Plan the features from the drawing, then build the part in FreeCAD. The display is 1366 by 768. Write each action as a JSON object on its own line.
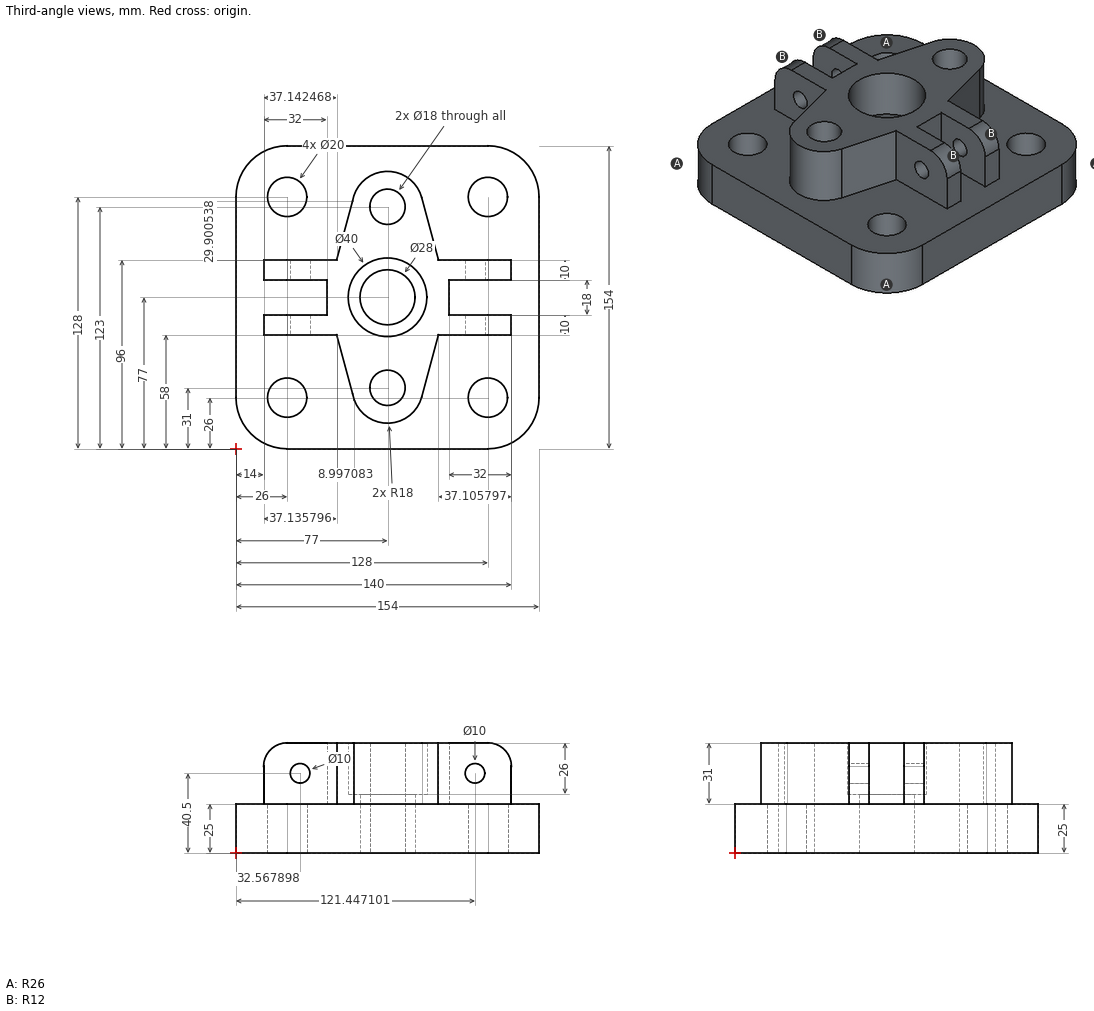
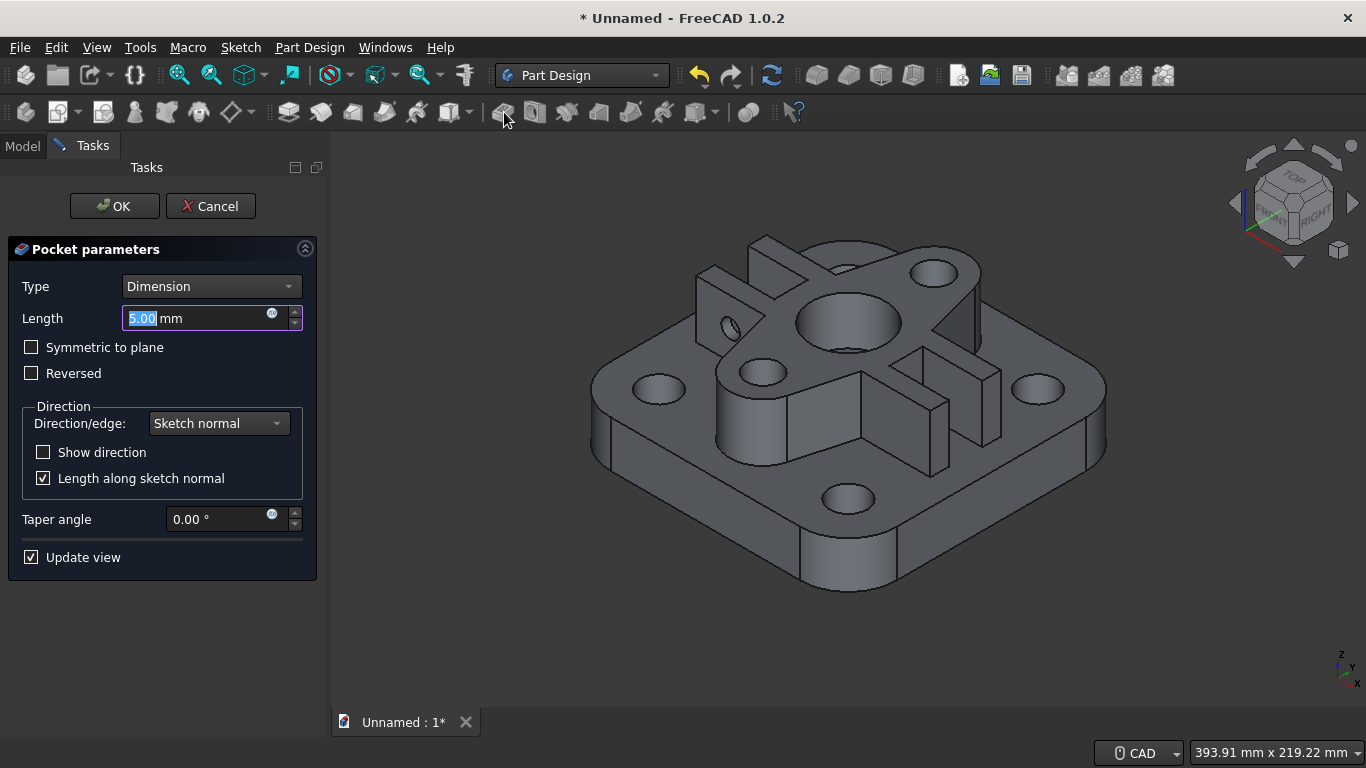
{"action": "left_click", "coordinate": [212, 286]}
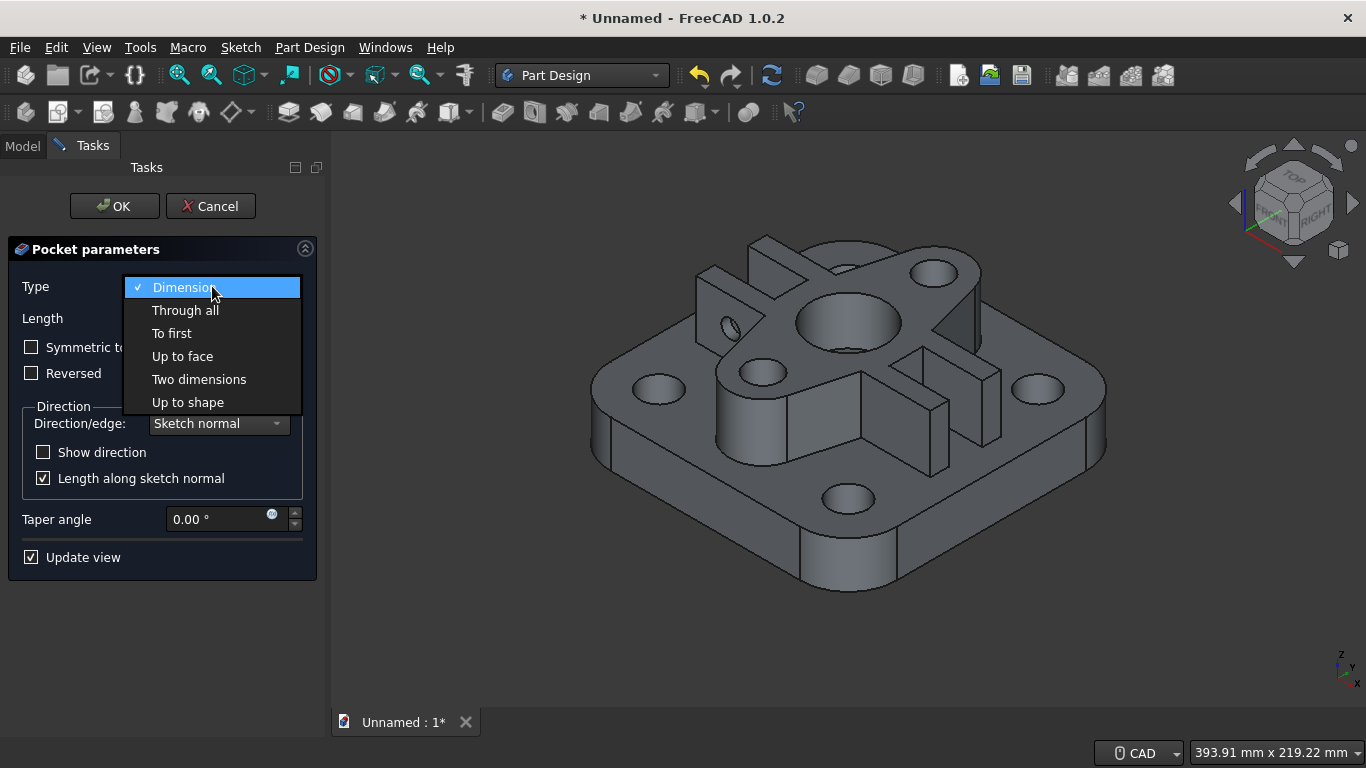
{"action": "left_click", "coordinate": [212, 310]}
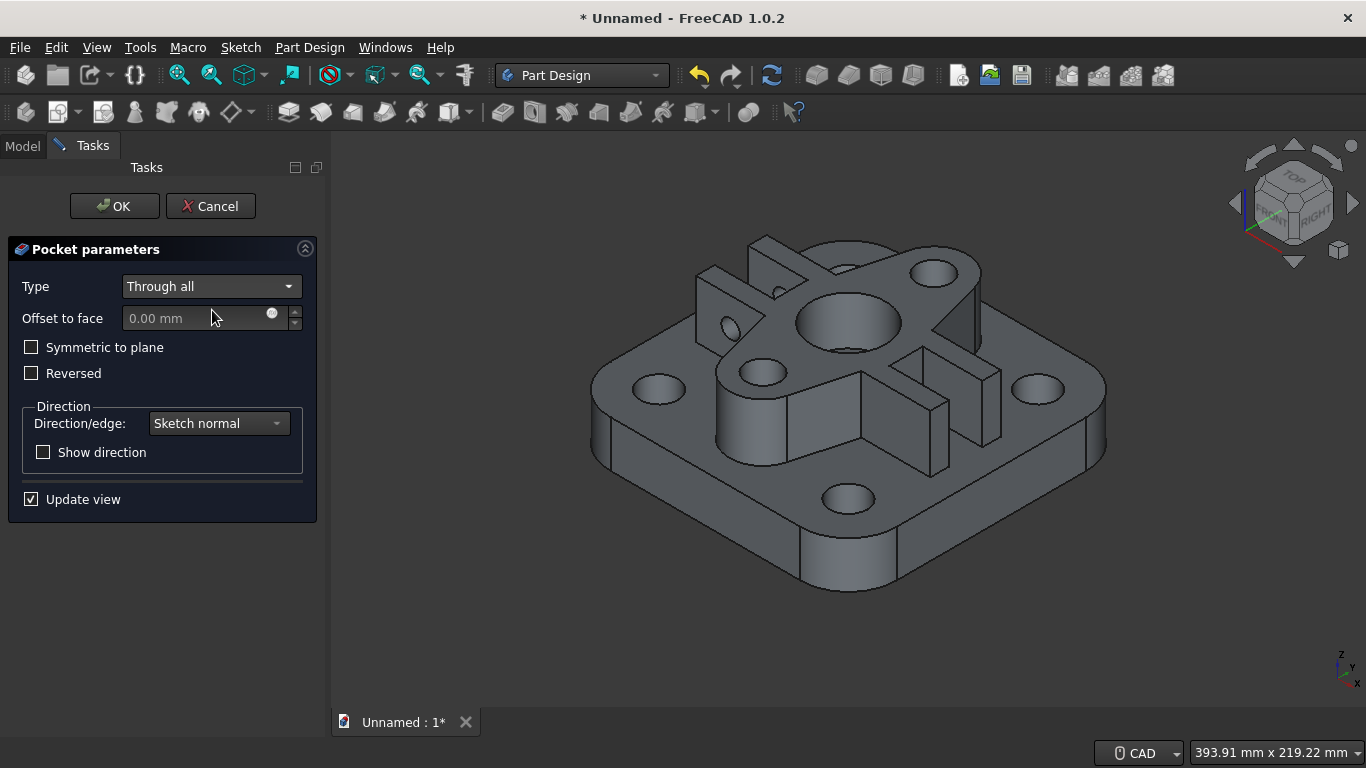
{"action": "left_click", "coordinate": [115, 206]}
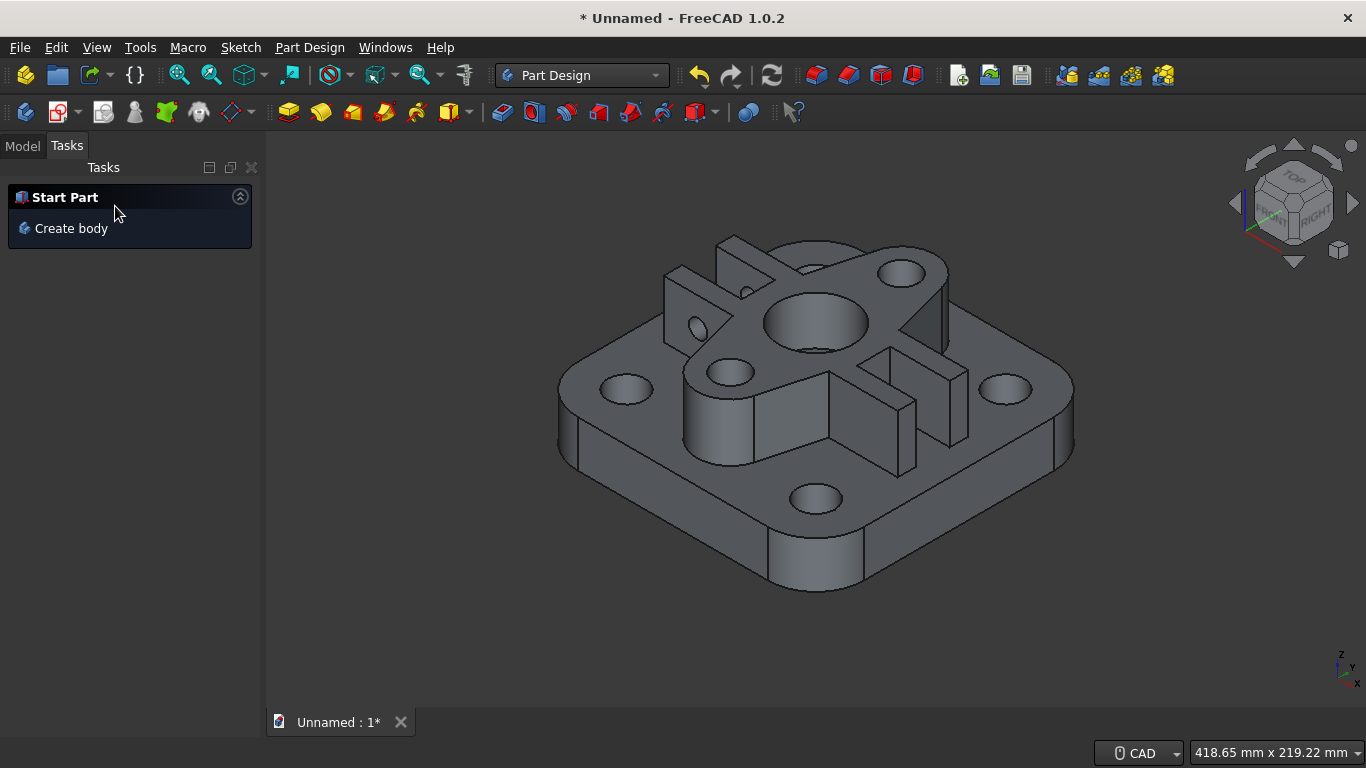
{"action": "left_click", "coordinate": [863, 423]}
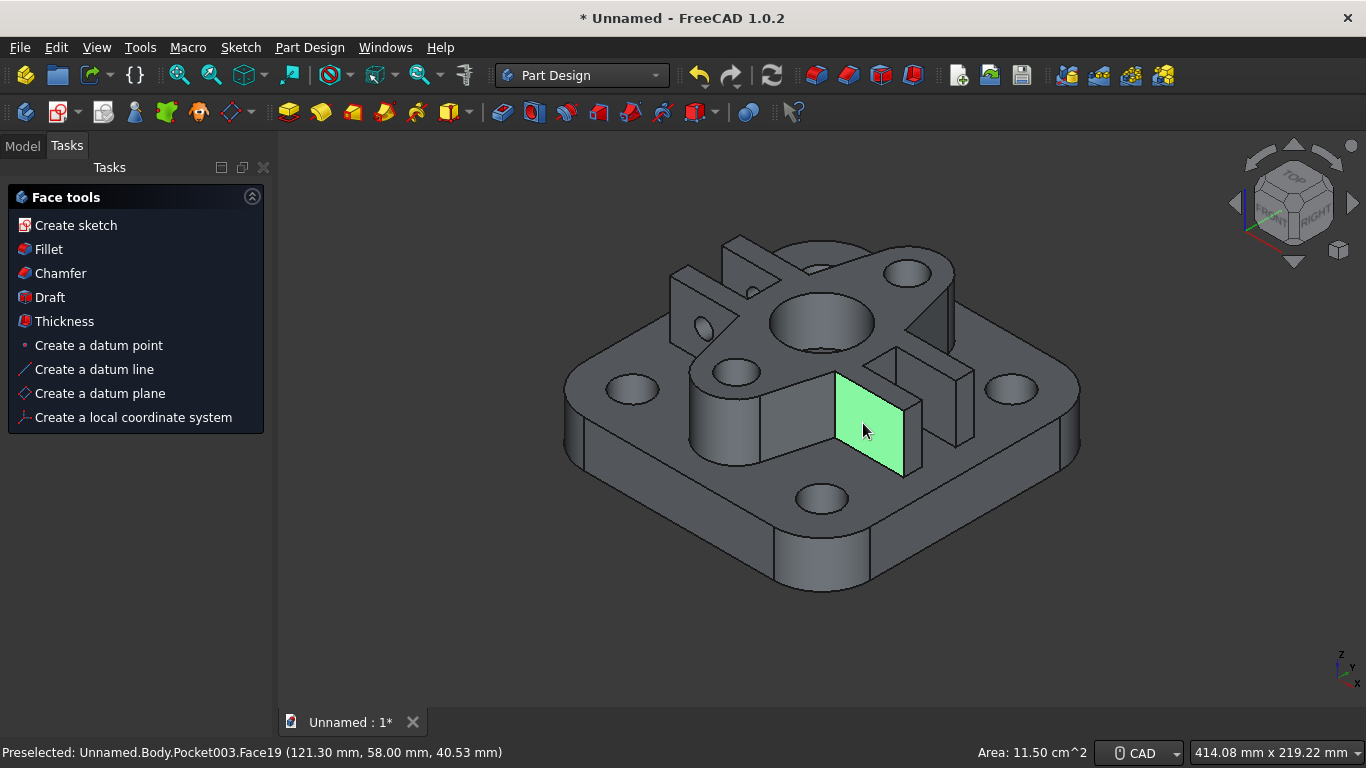
{"action": "left_click", "coordinate": [58, 112]}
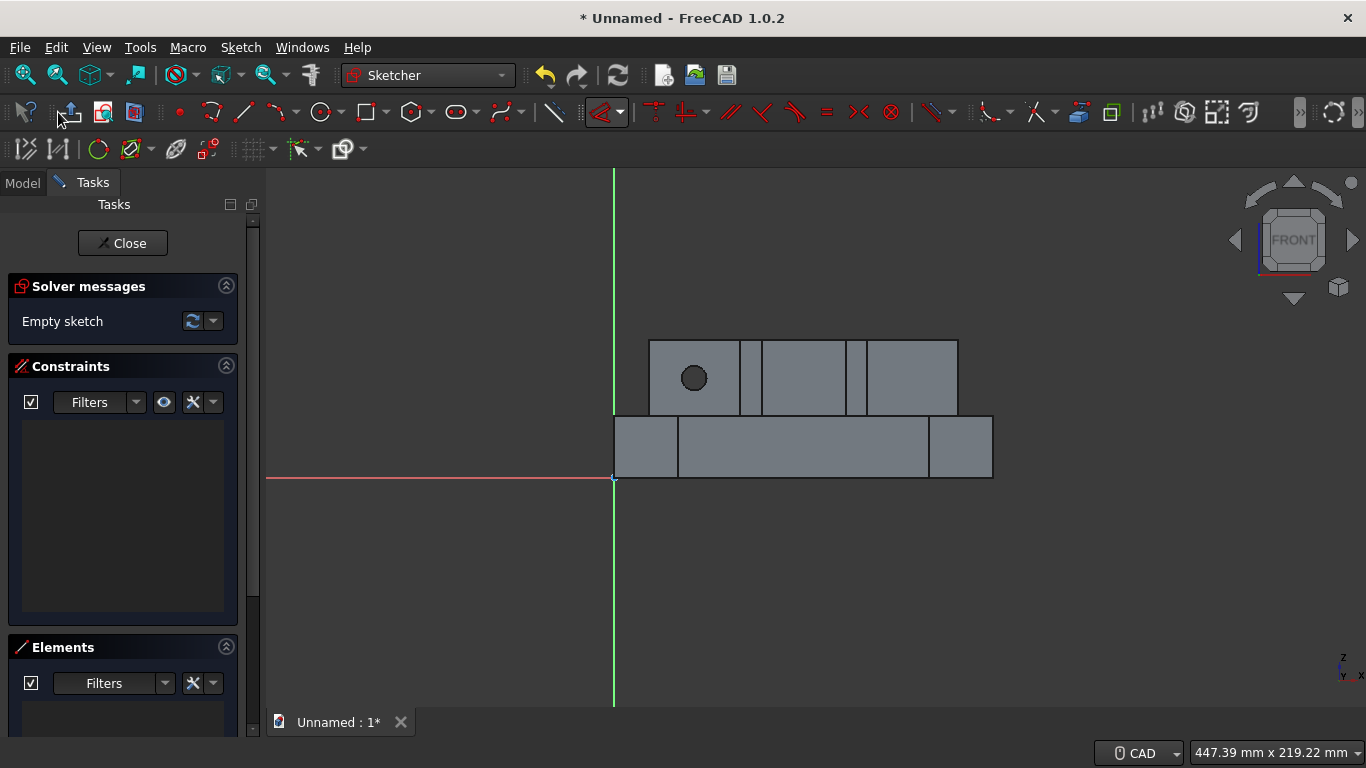
{"action": "left_click", "coordinate": [136, 112]}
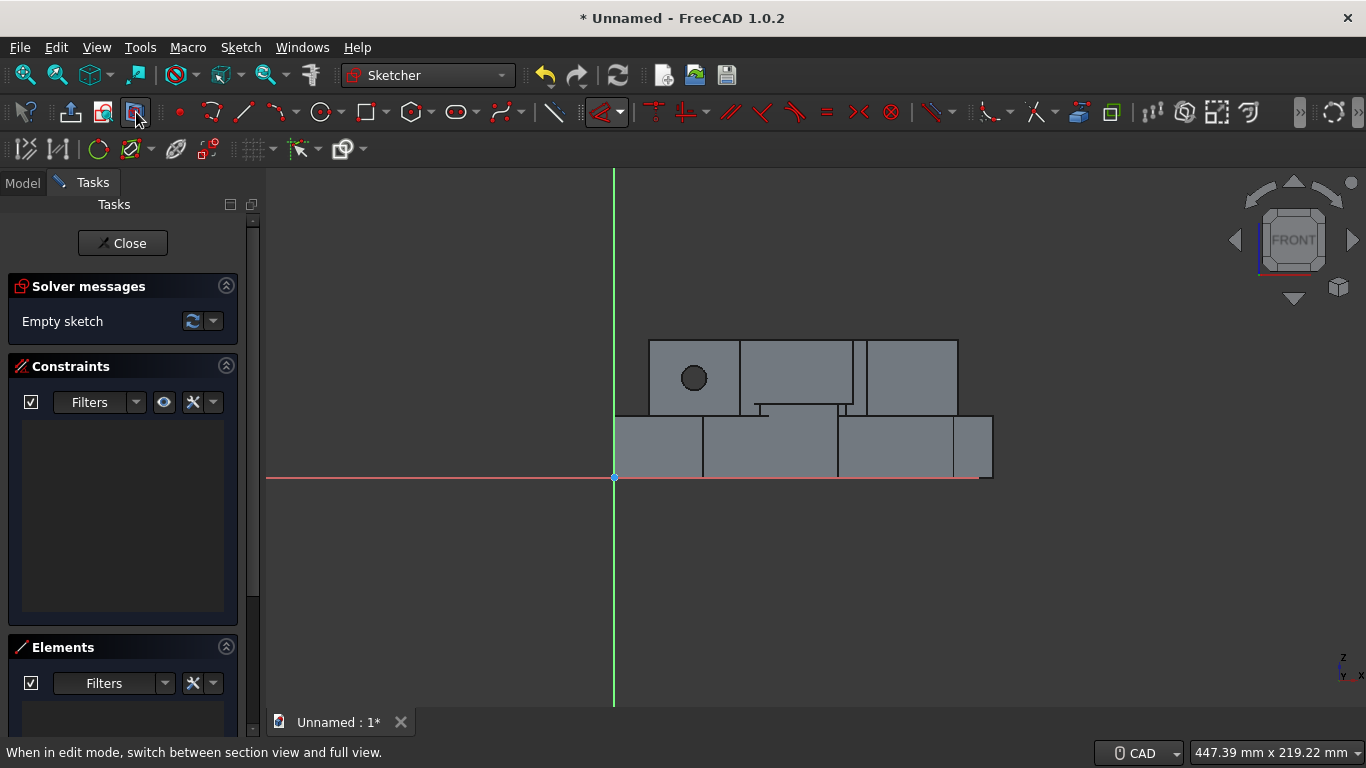
{"action": "scroll", "coordinate": [926, 373], "scroll_direction": "up", "scroll_amount": 13}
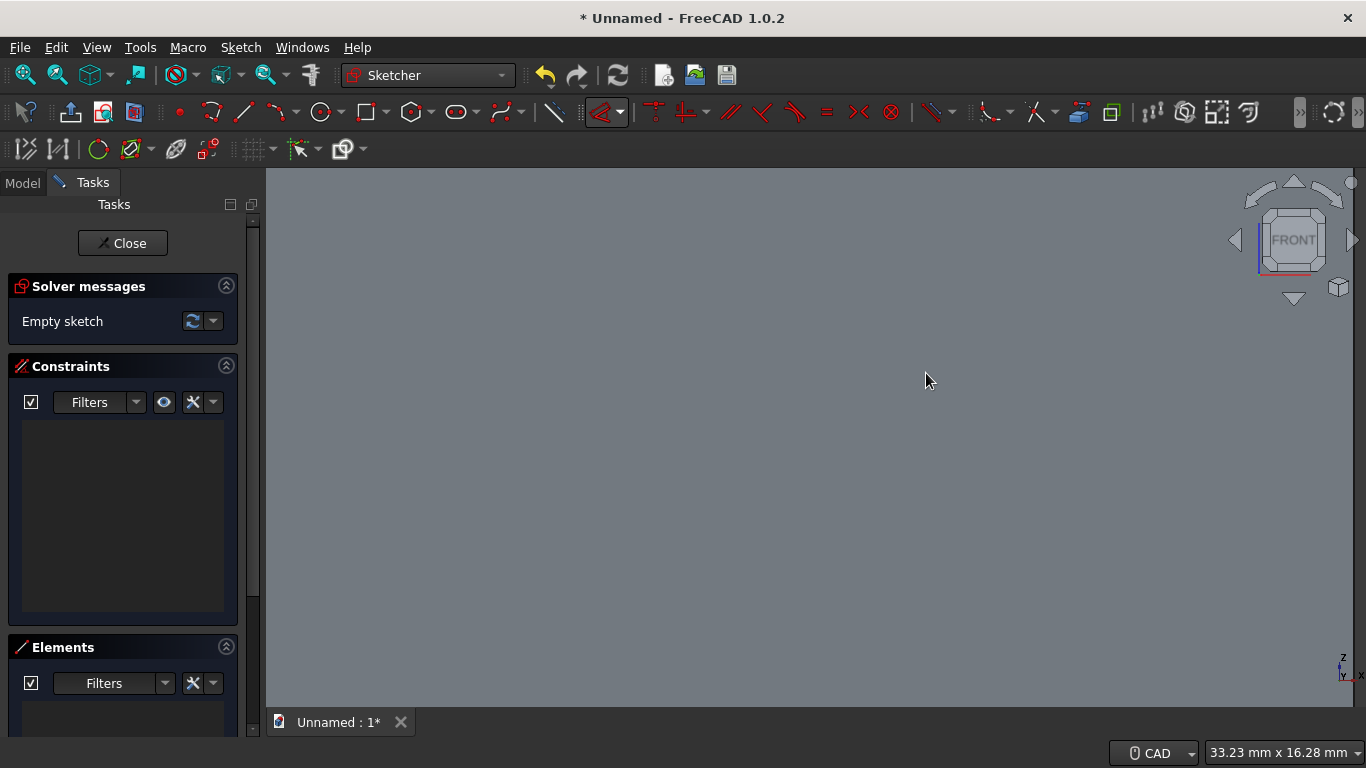
{"action": "left_click", "coordinate": [322, 112]}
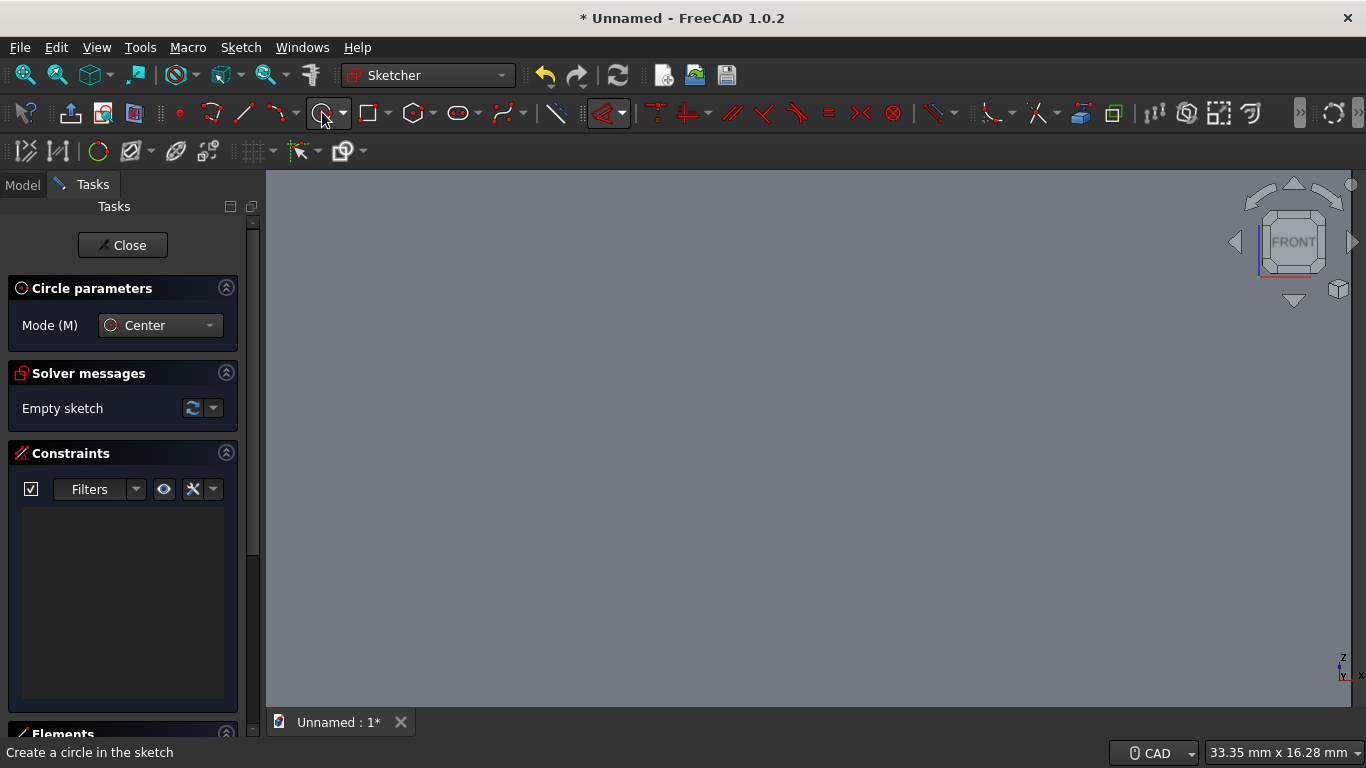
{"action": "left_click", "coordinate": [740, 437]}
{"action": "left_click", "coordinate": [857, 321]}
{"action": "key", "text": "Escape"}